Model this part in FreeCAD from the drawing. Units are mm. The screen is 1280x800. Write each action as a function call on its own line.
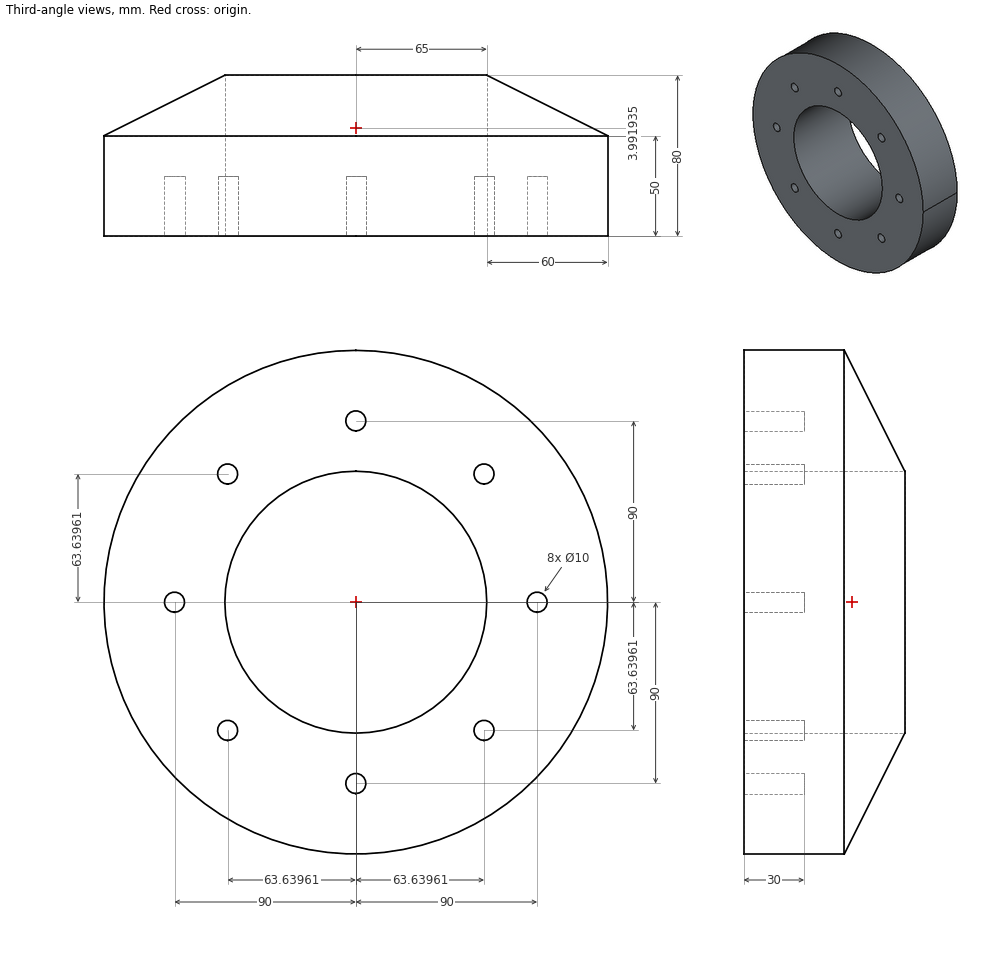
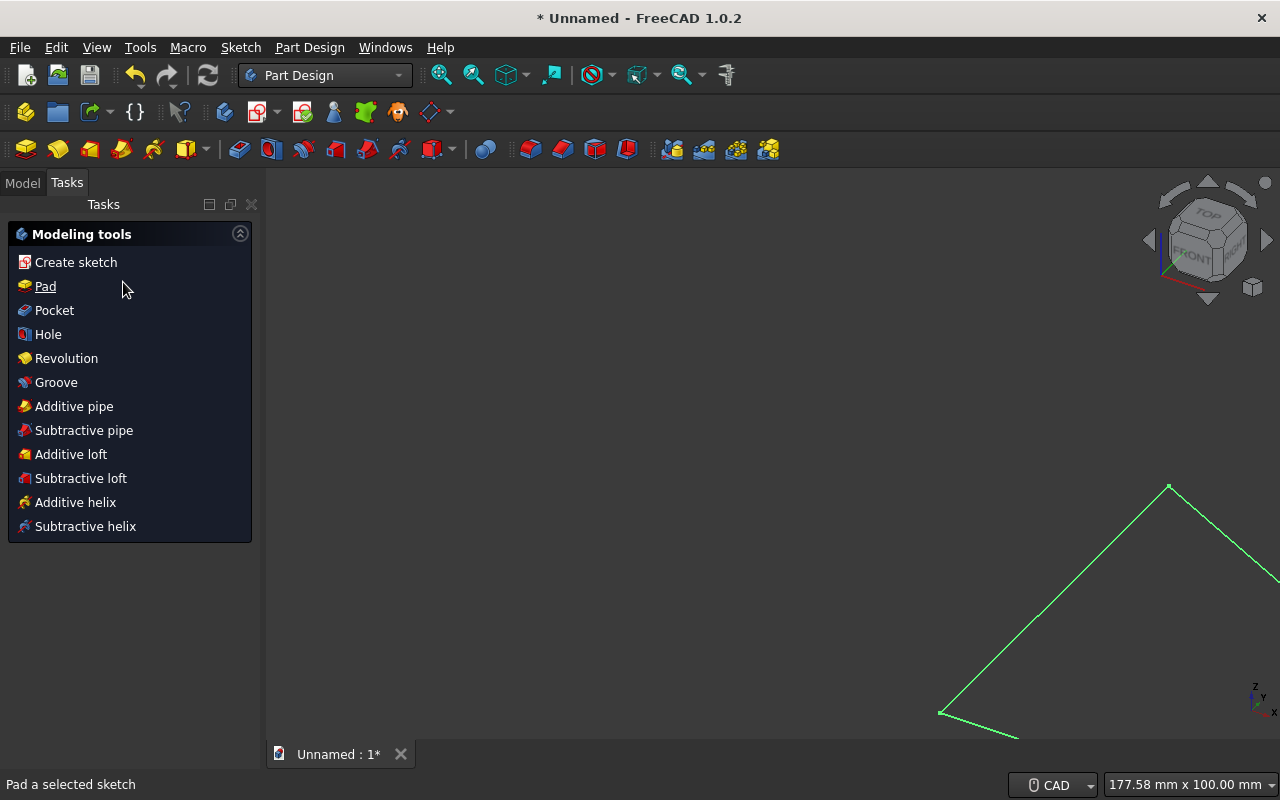
click(58, 150)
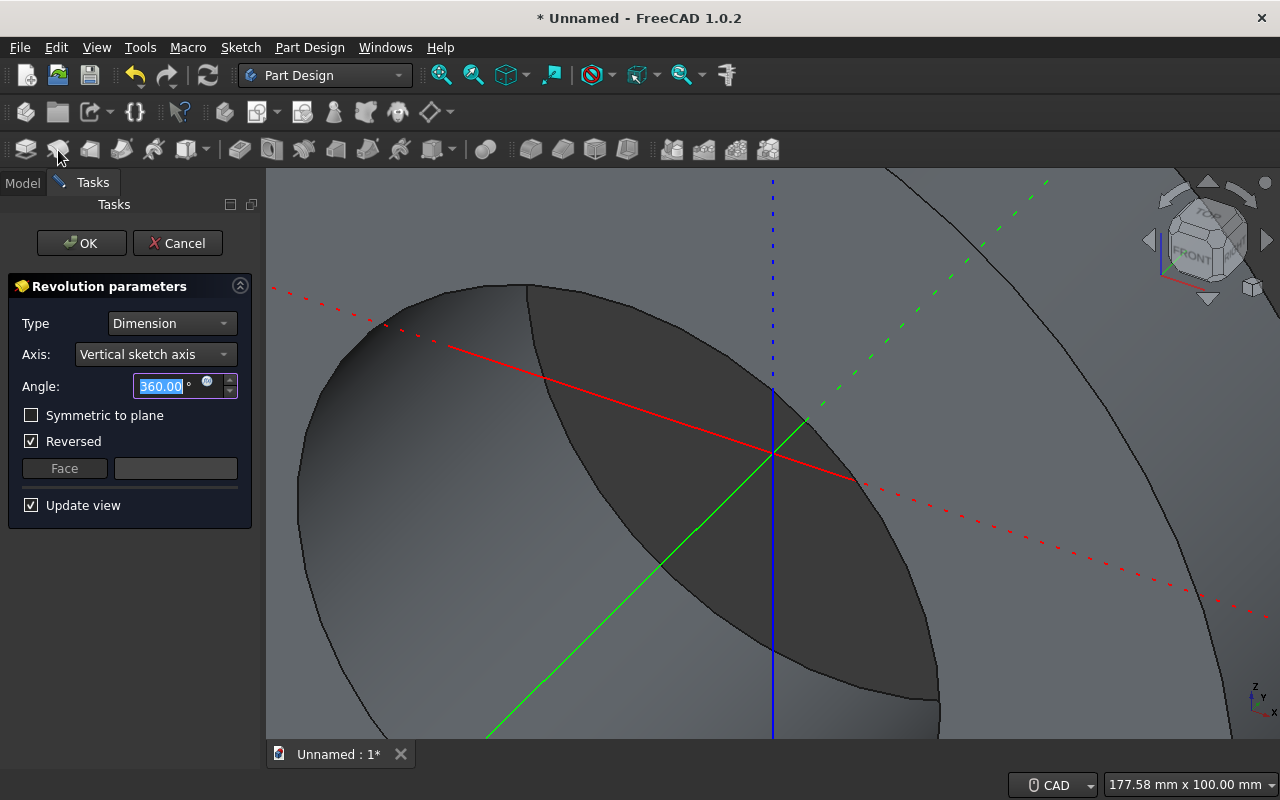
click(82, 243)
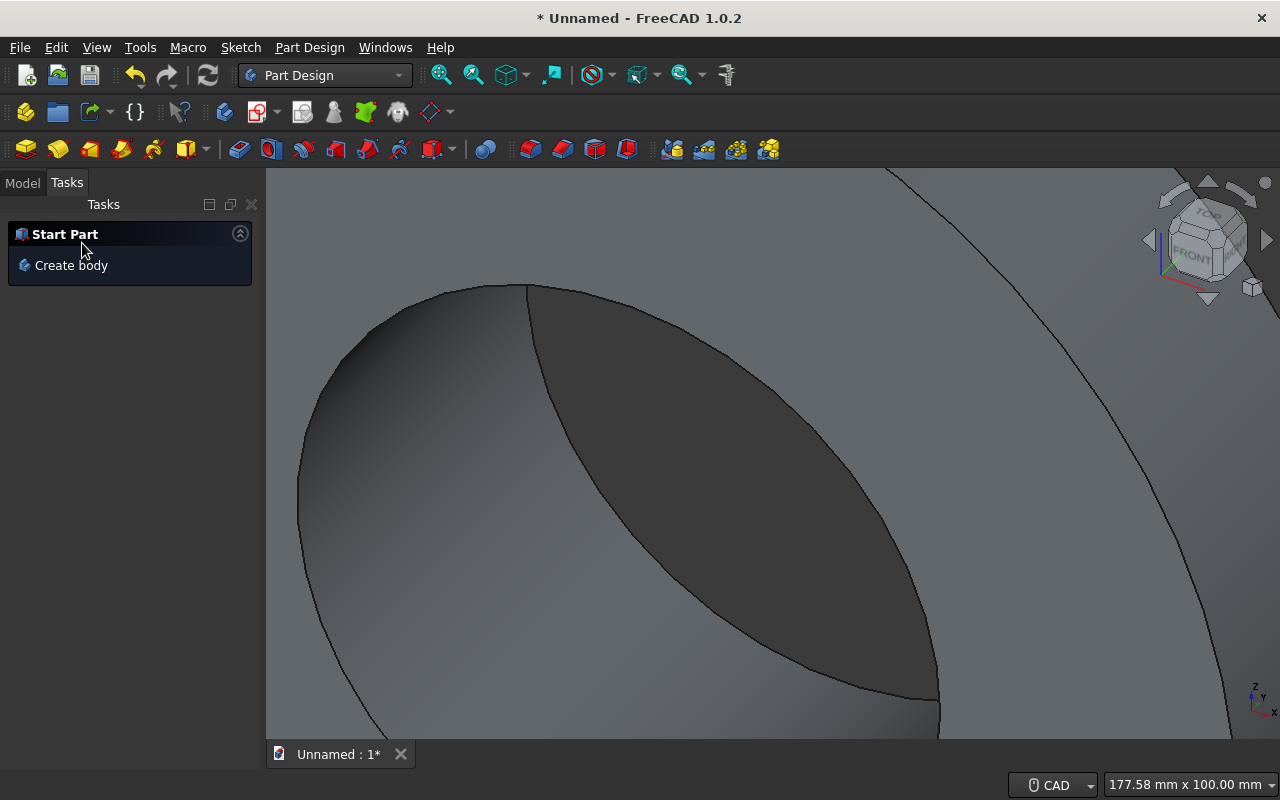
click(442, 76)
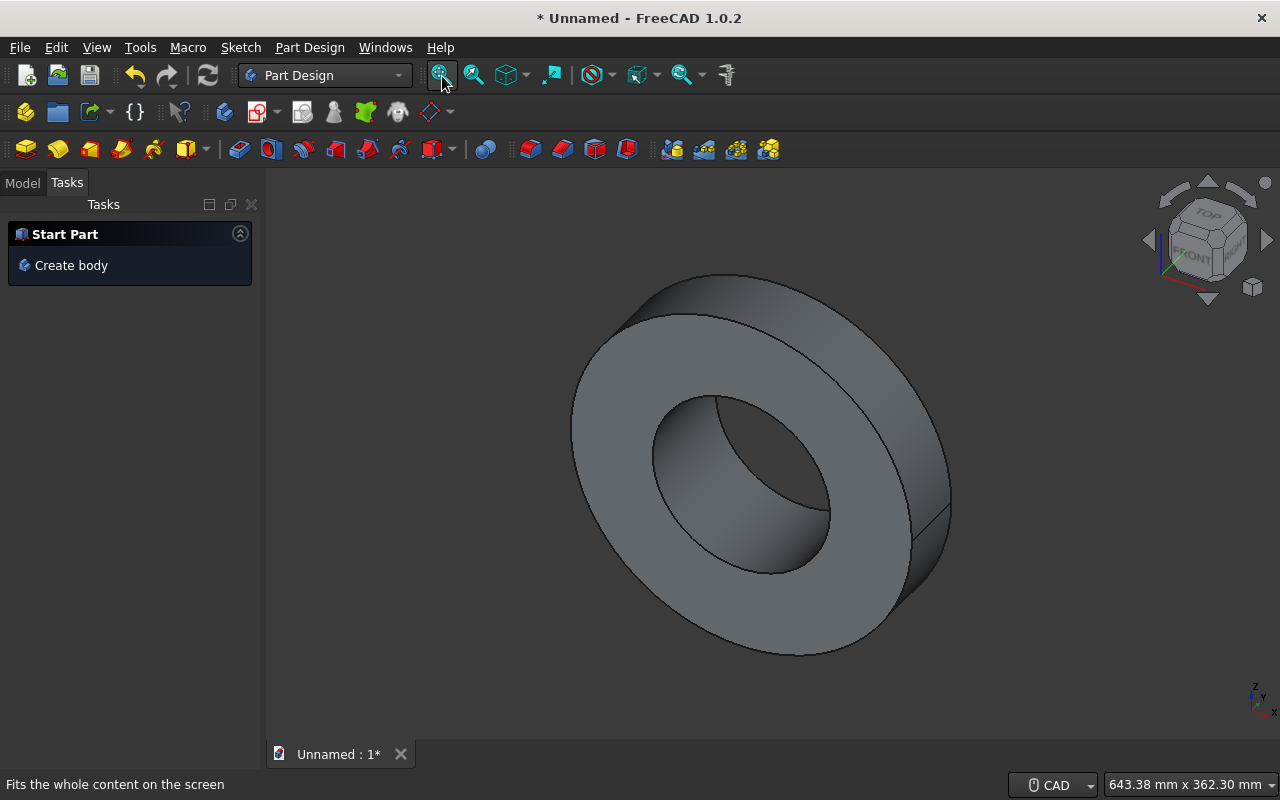
click(644, 359)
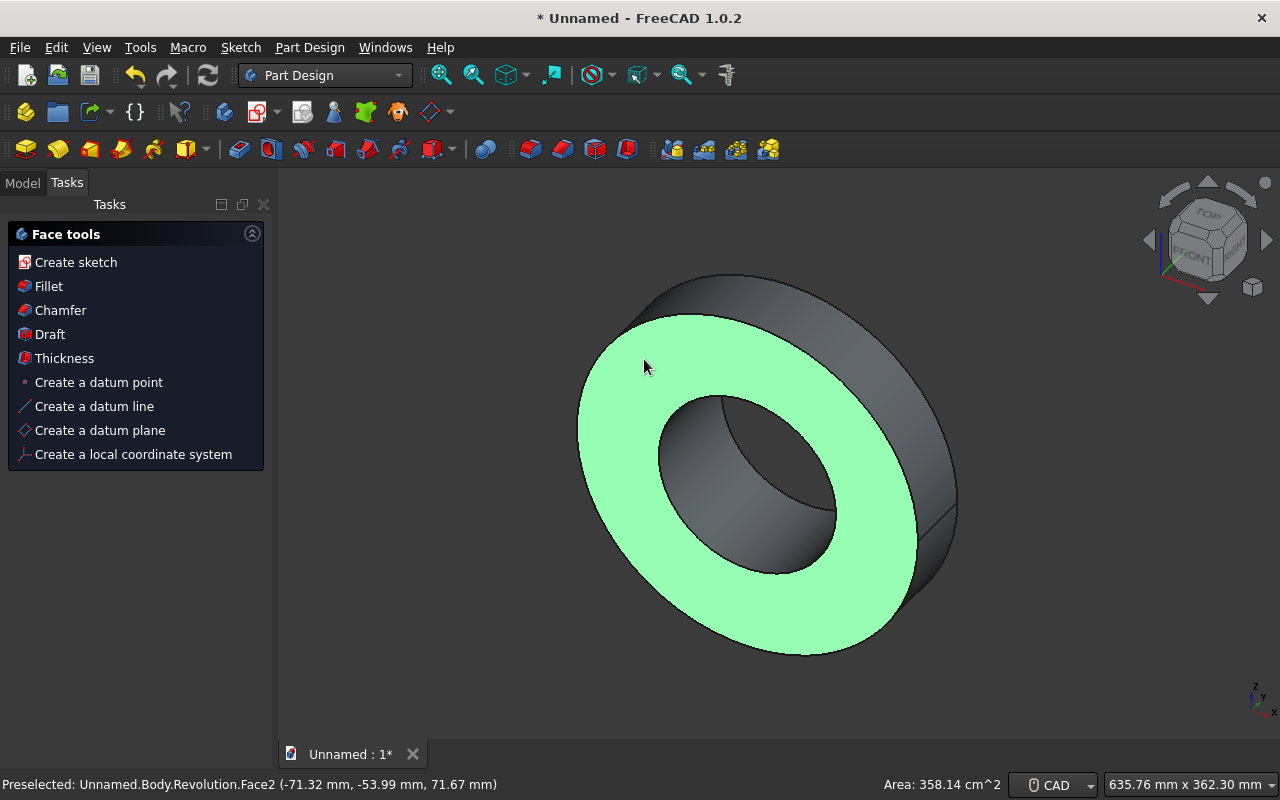
click(258, 112)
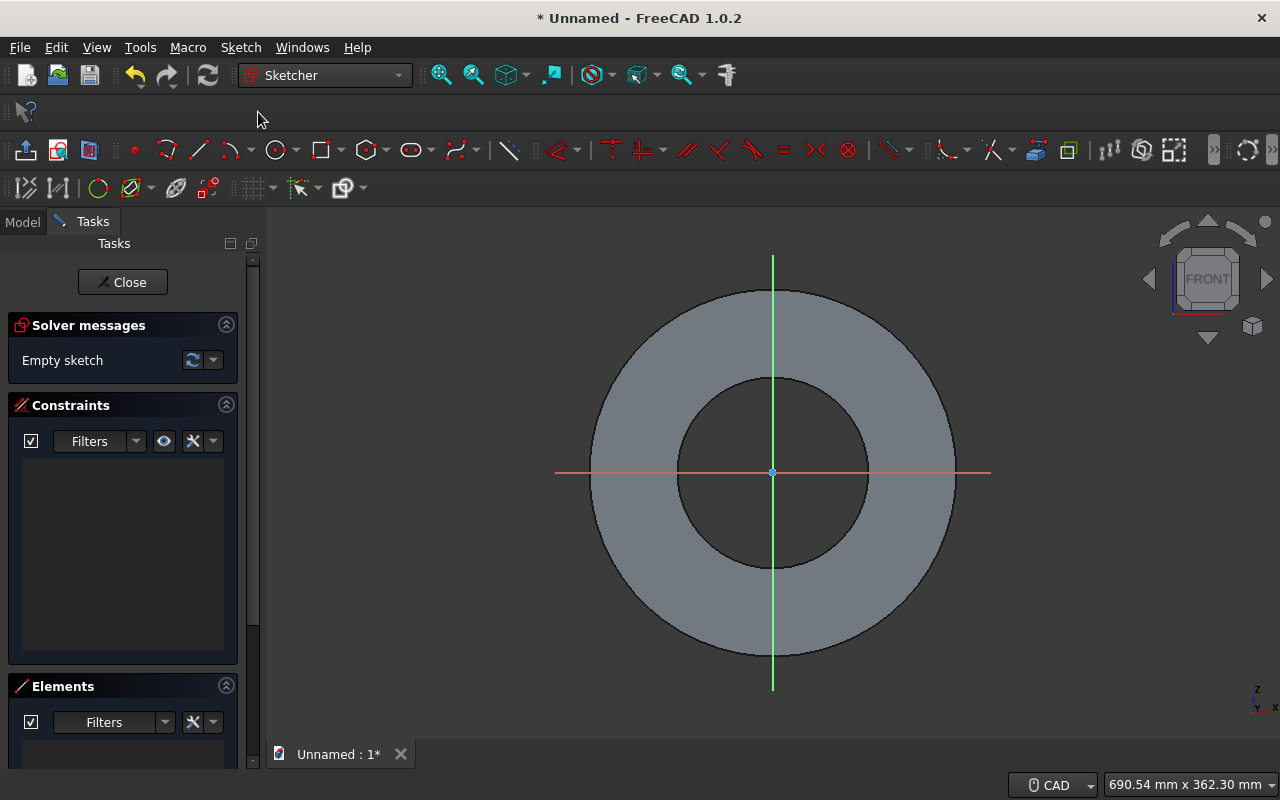
click(276, 150)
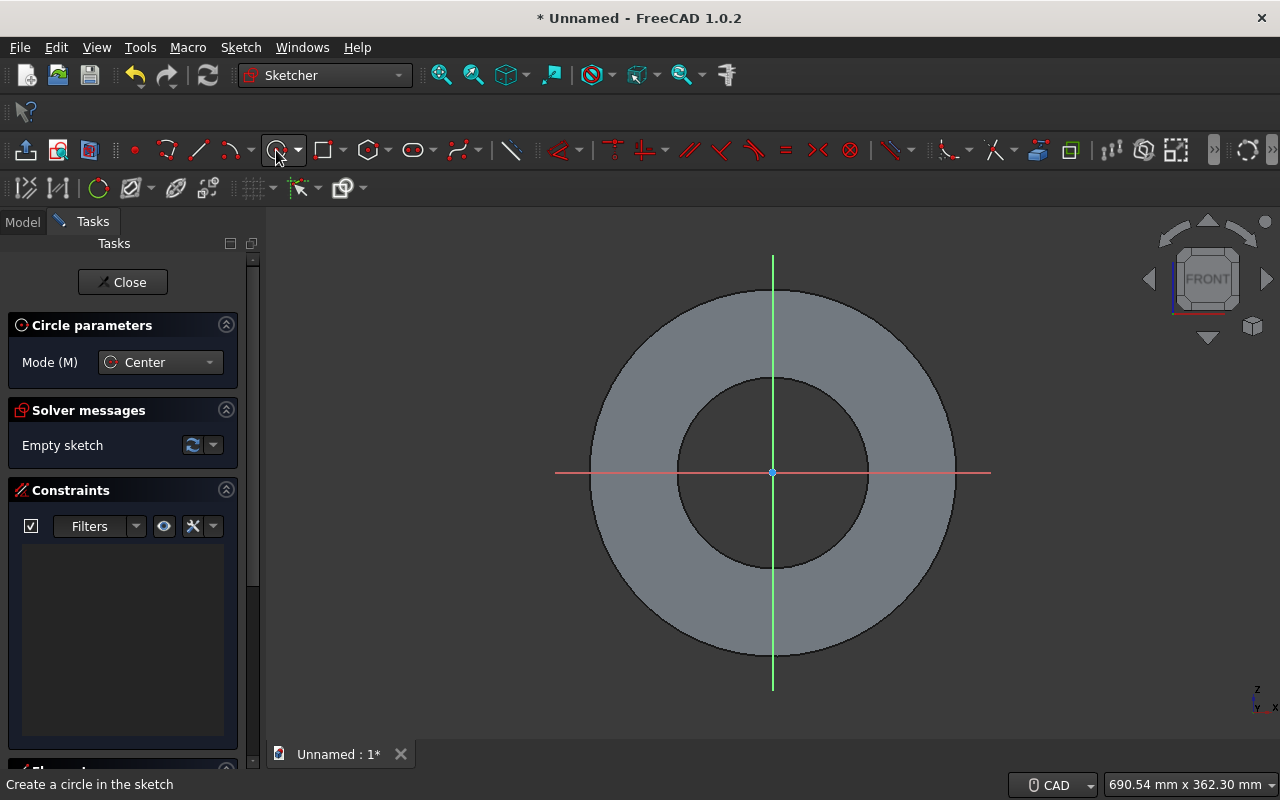
scroll(905, 473, up, 6)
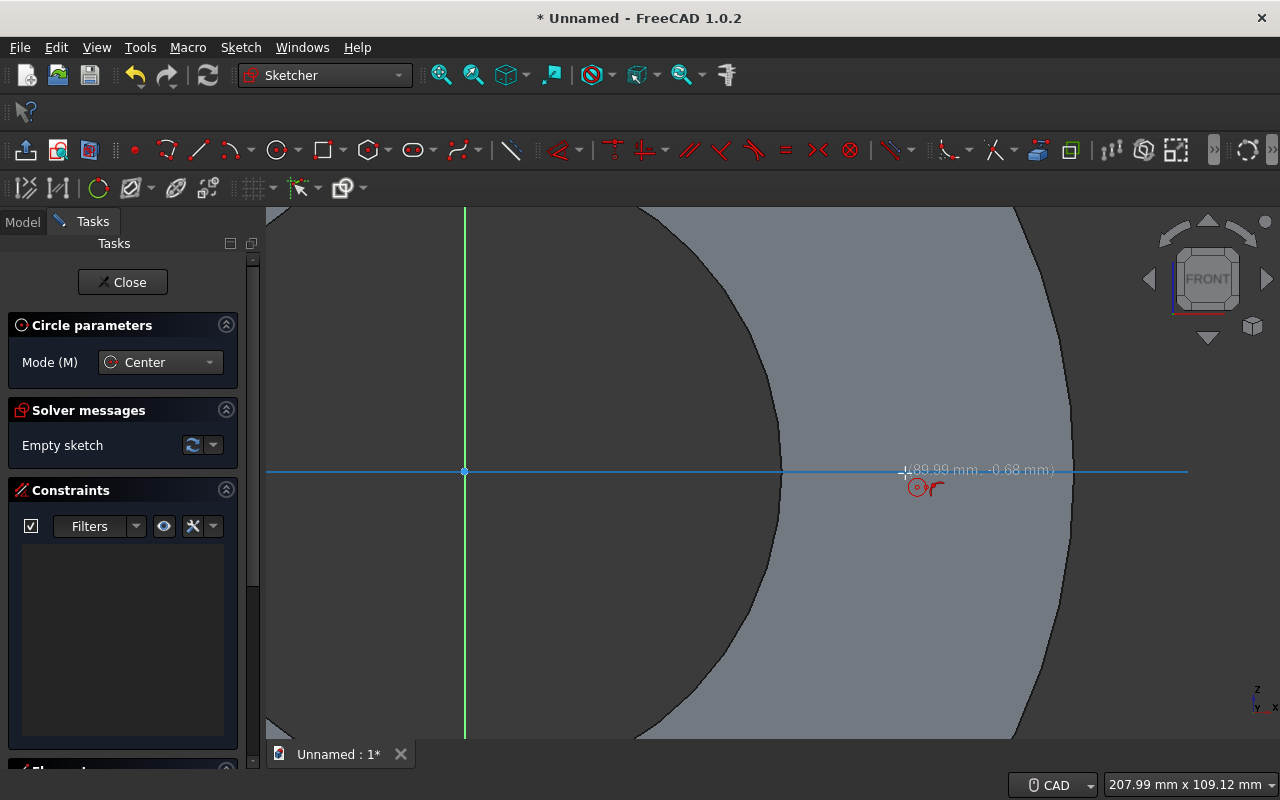
click(904, 472)
click(921, 455)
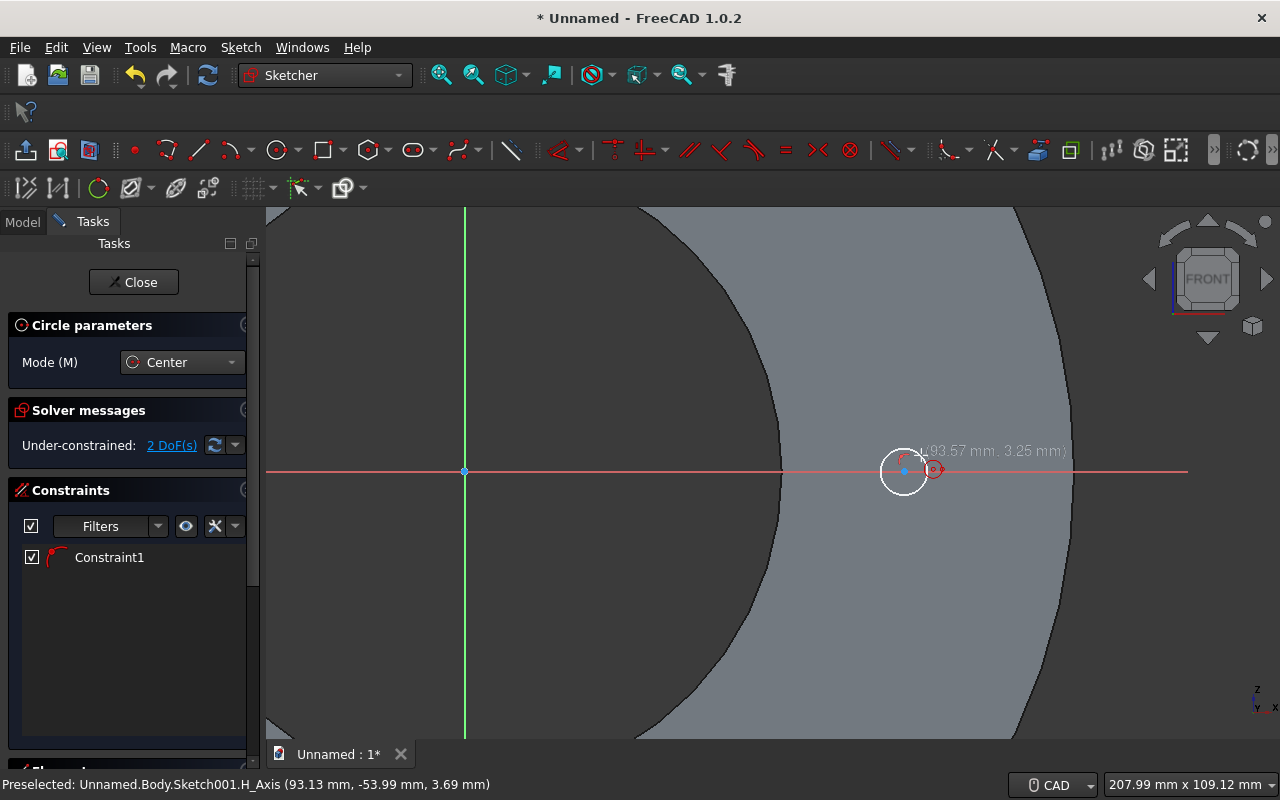
scroll(844, 474, down, 5)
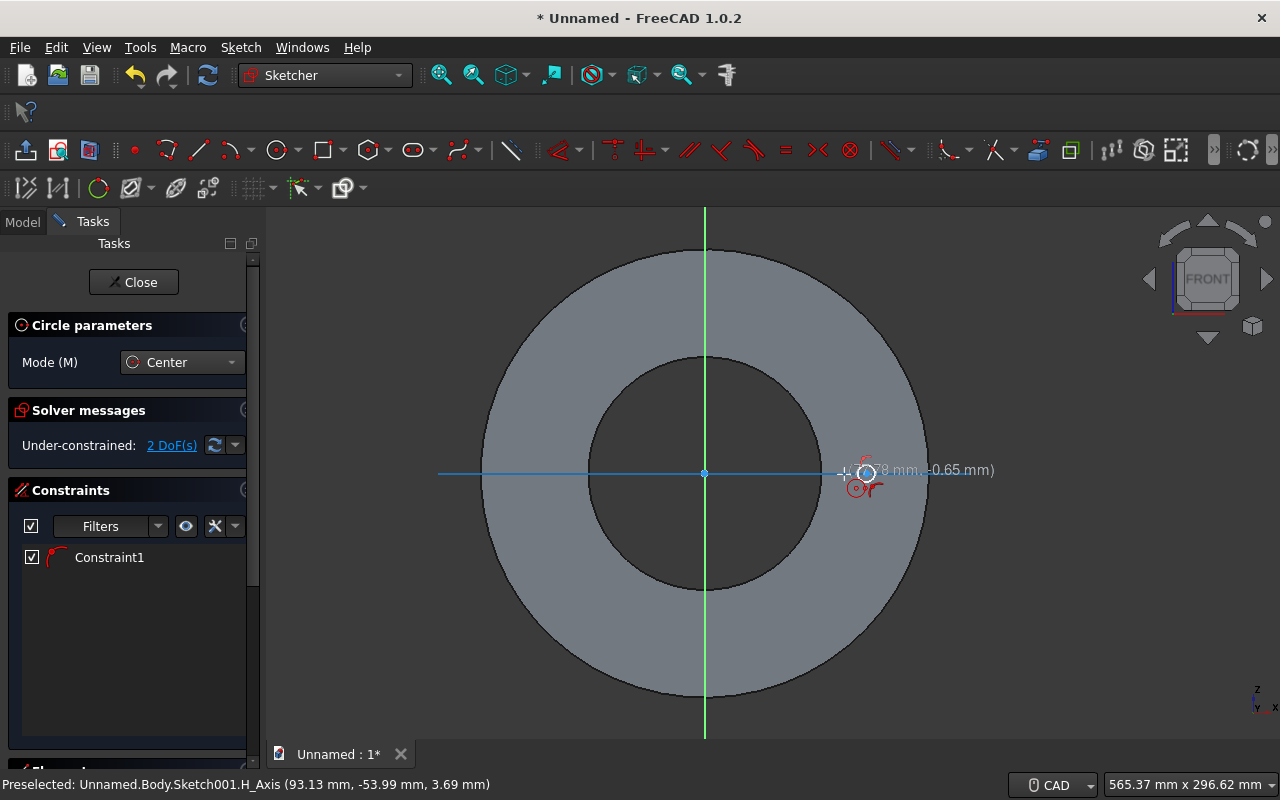
scroll(819, 588, up, 5)